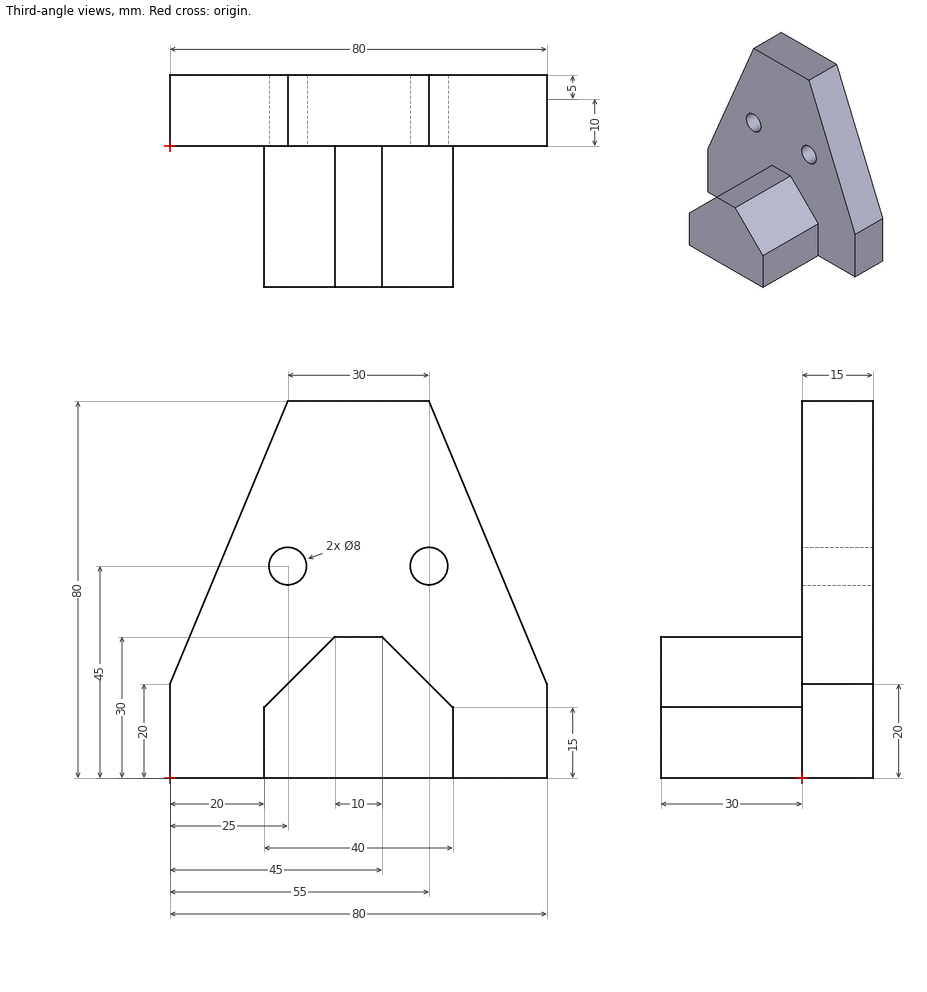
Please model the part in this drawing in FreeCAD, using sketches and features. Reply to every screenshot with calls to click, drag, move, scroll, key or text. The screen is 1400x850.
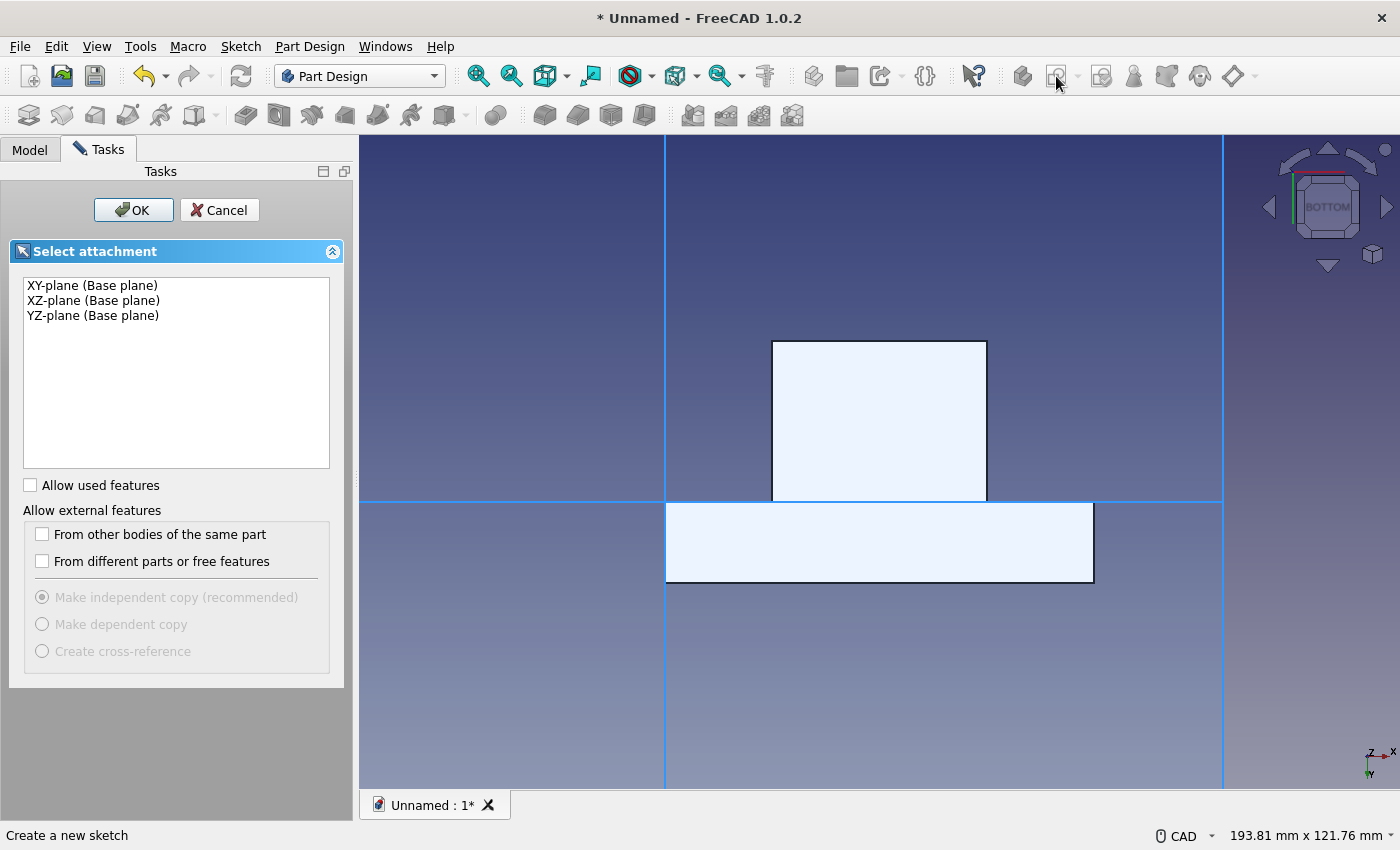
click(84, 300)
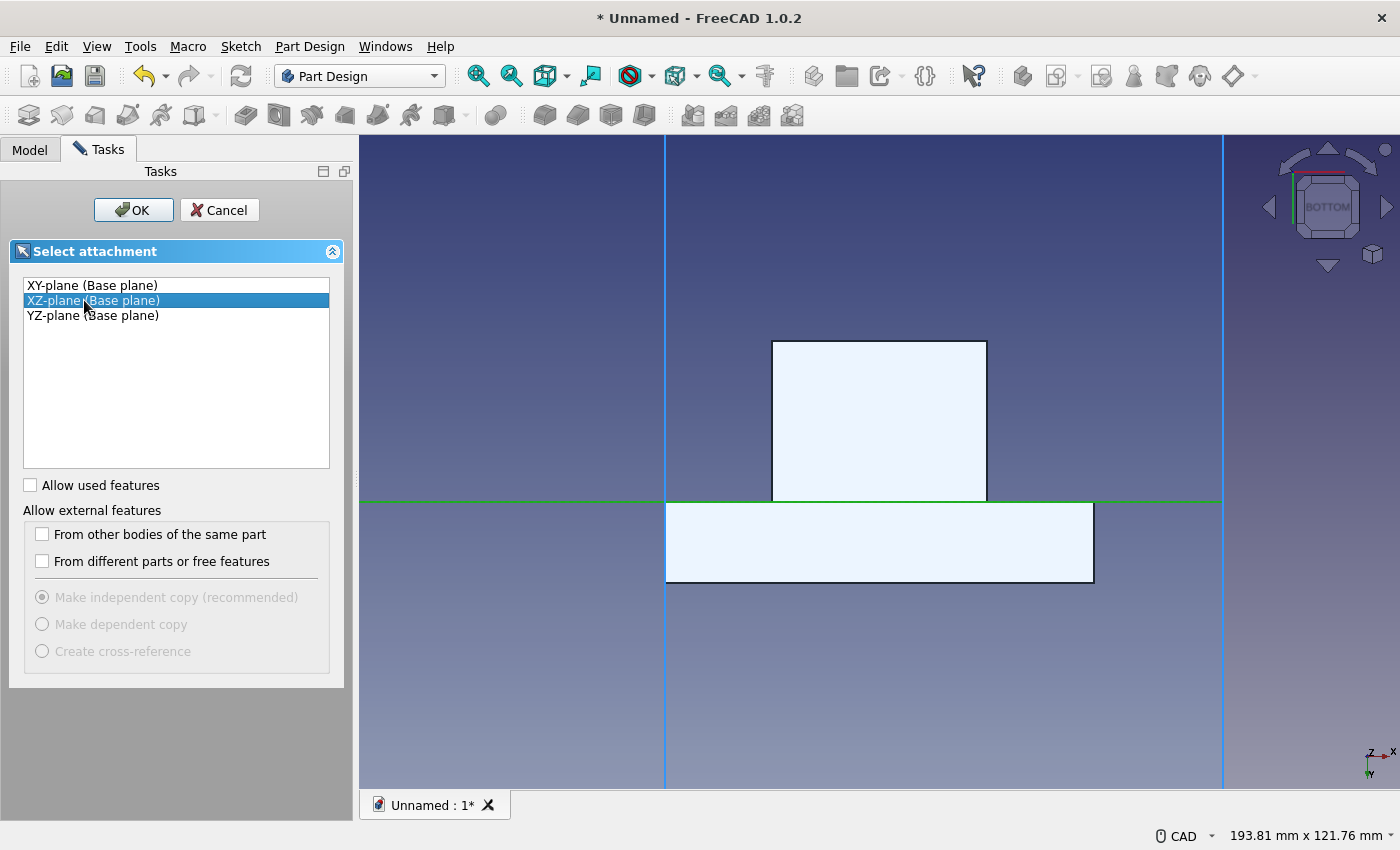
click(134, 210)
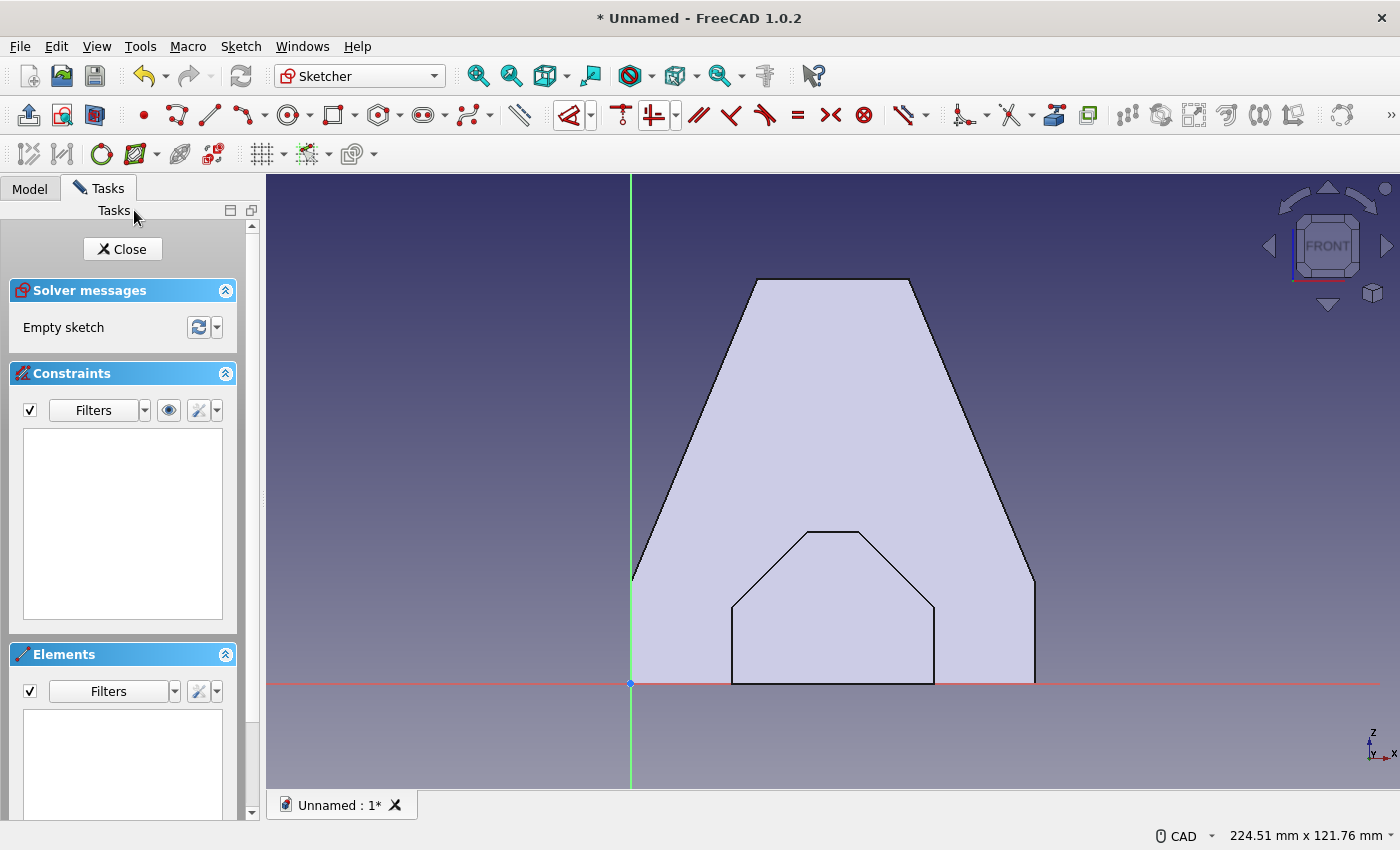
click(95, 116)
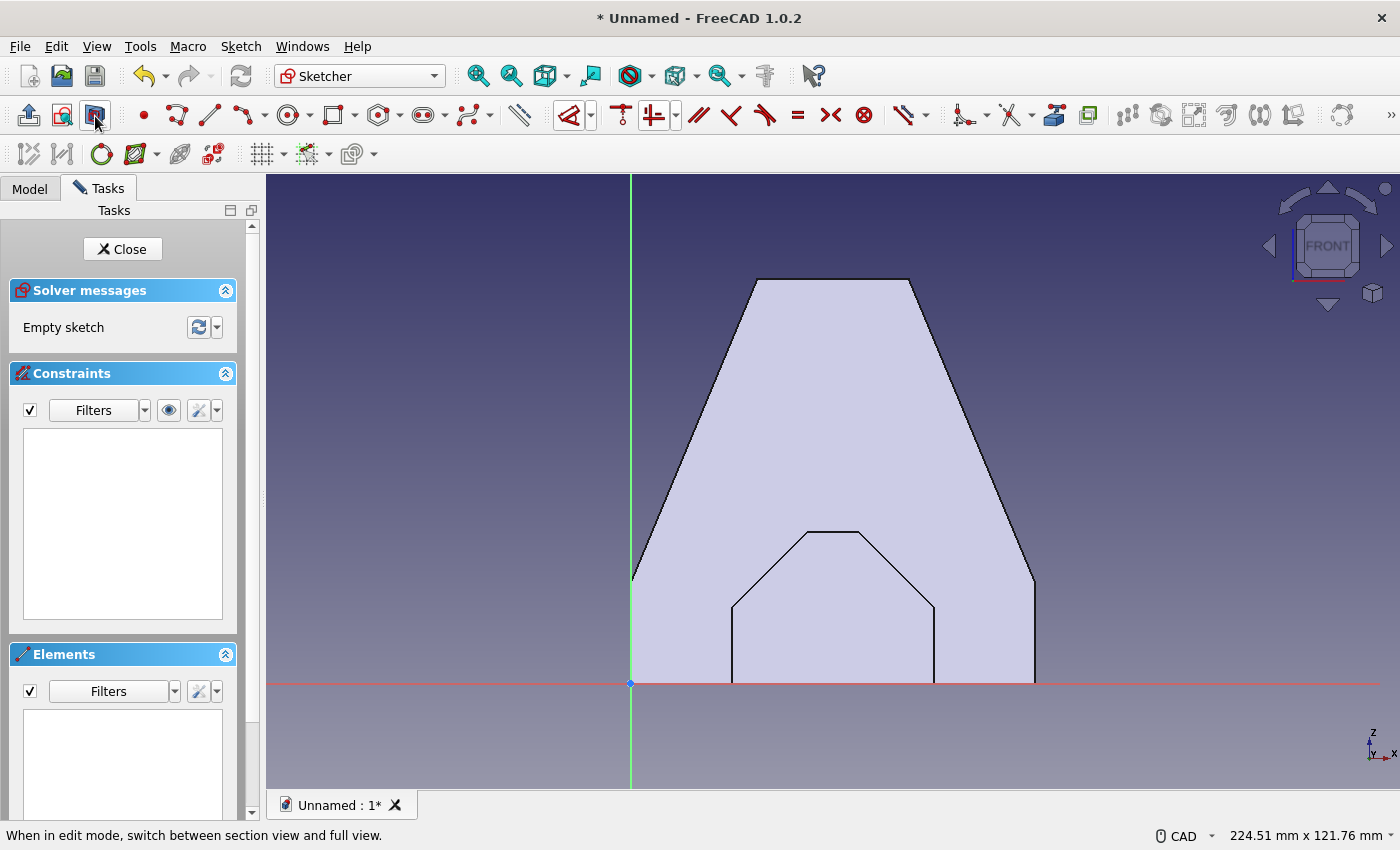
scroll(811, 719, up, 2)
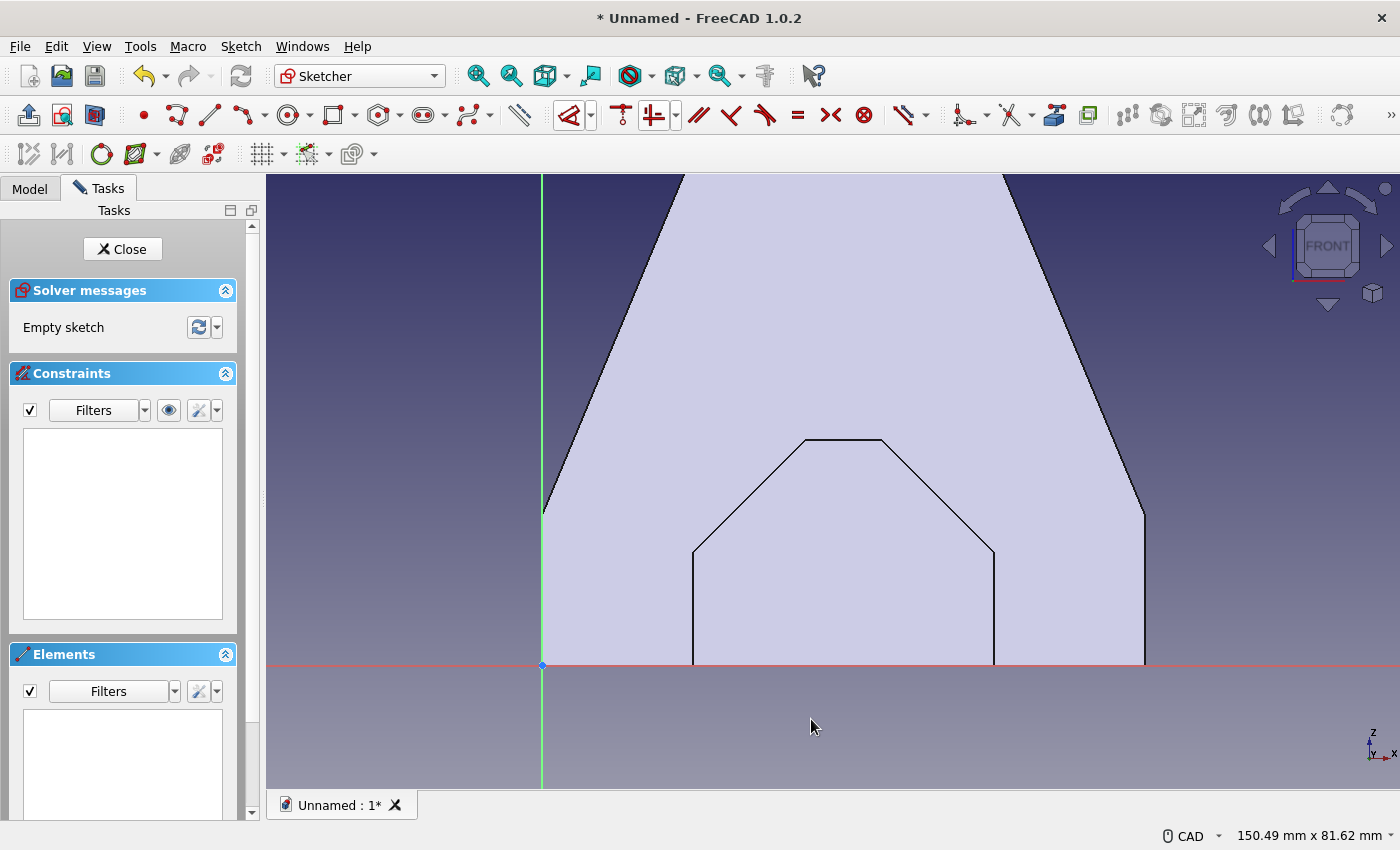
key(g)
key(c)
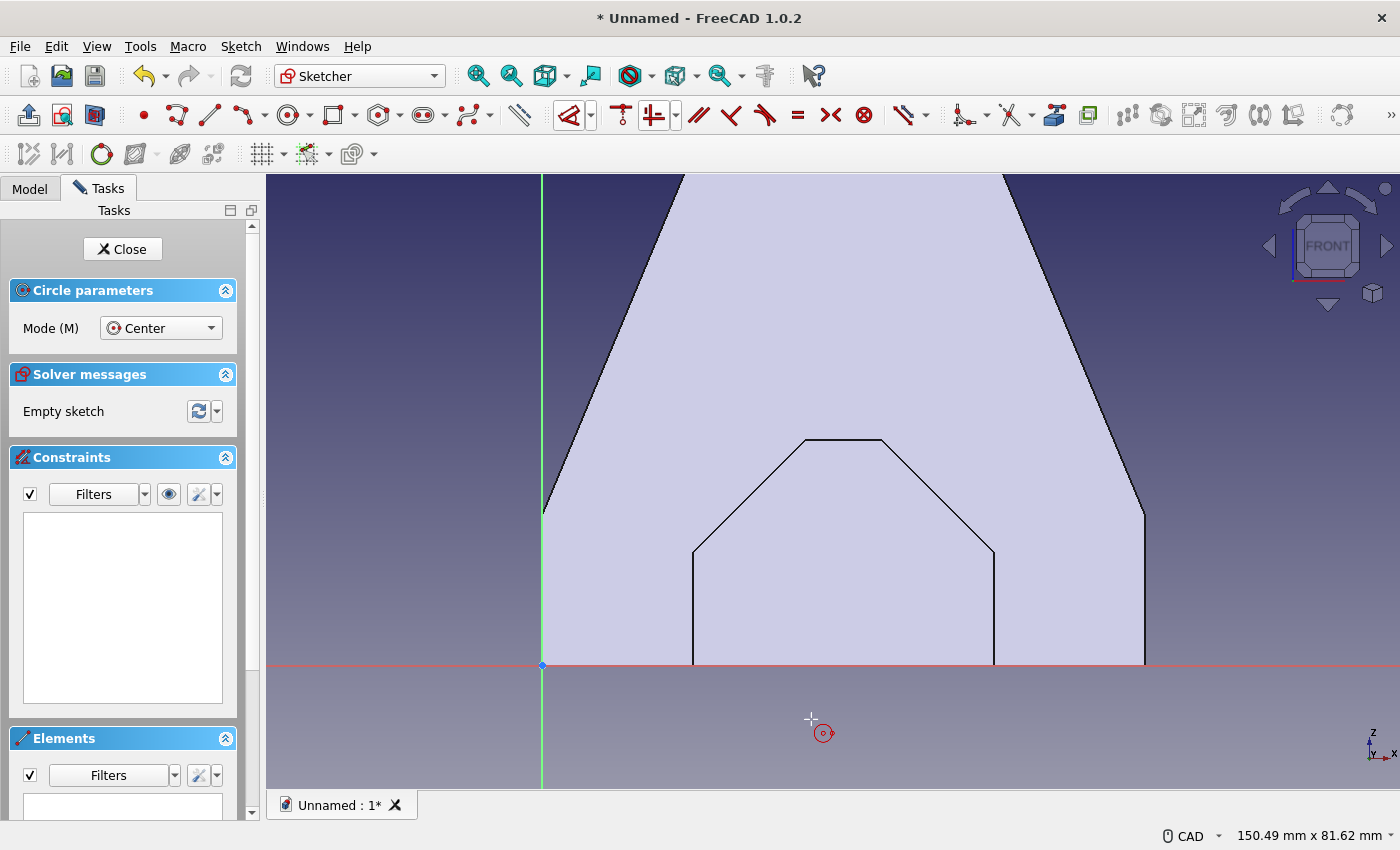
click(731, 327)
move(752, 305)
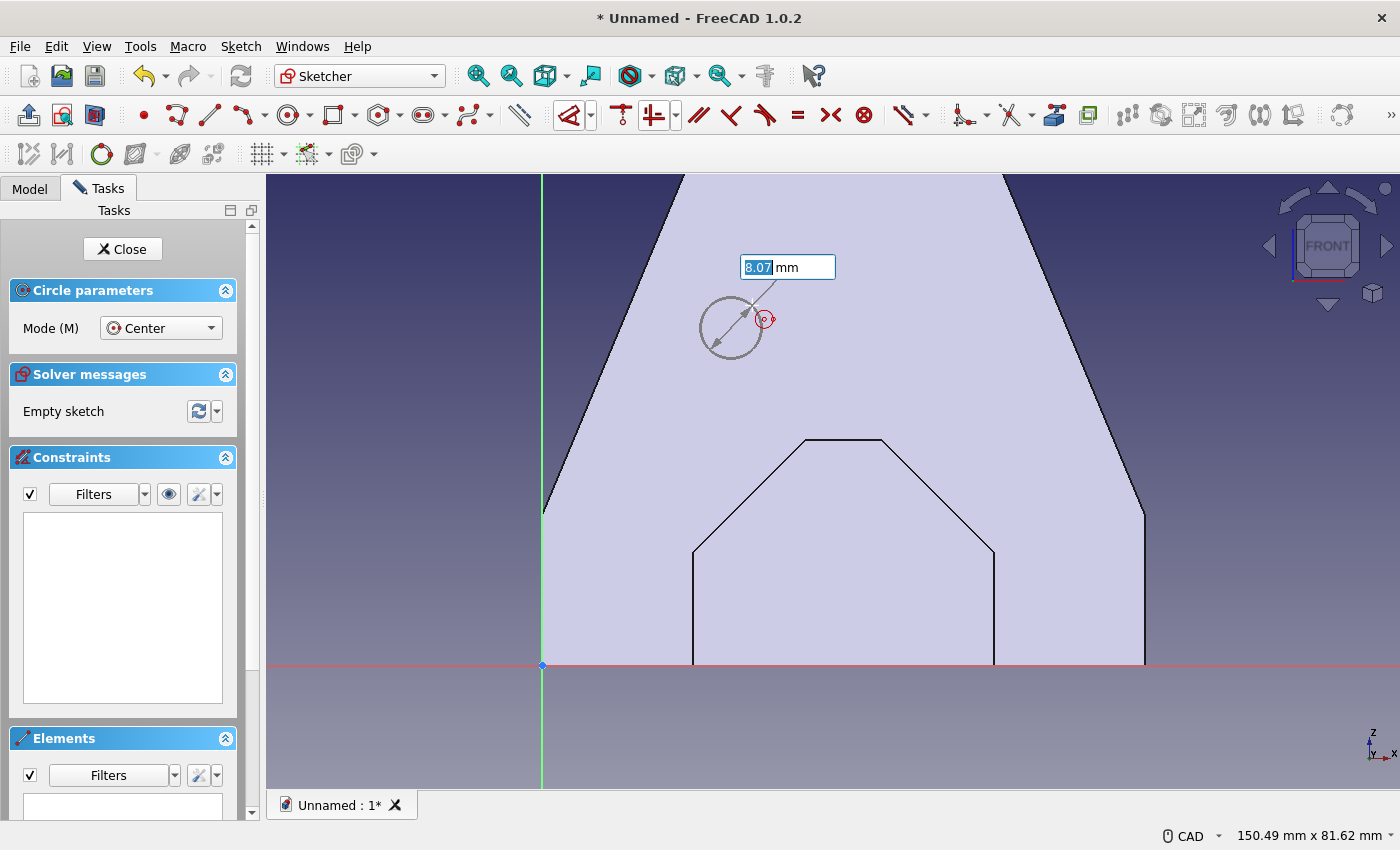
text(8)
key(Return)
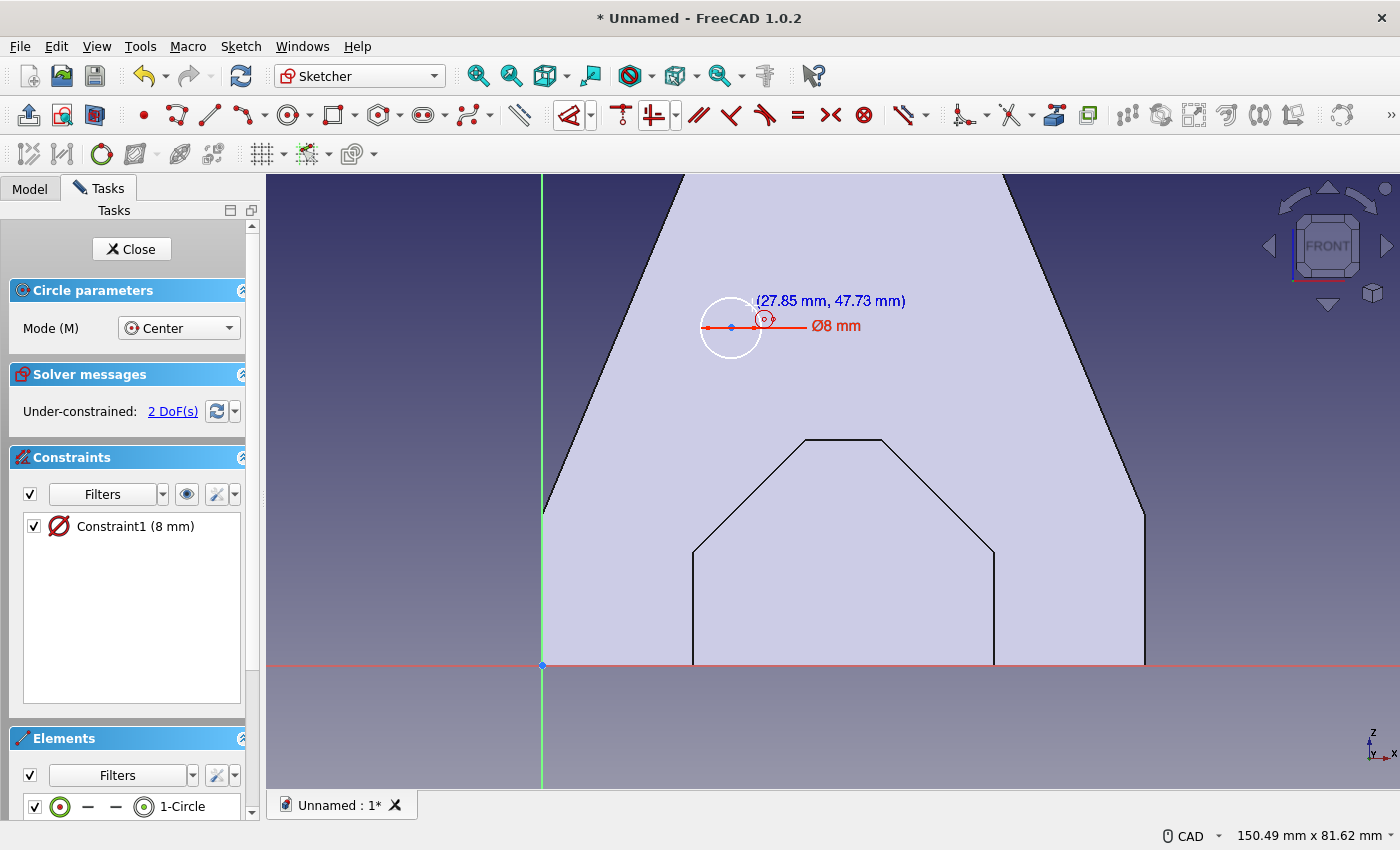
click(957, 327)
move(978, 305)